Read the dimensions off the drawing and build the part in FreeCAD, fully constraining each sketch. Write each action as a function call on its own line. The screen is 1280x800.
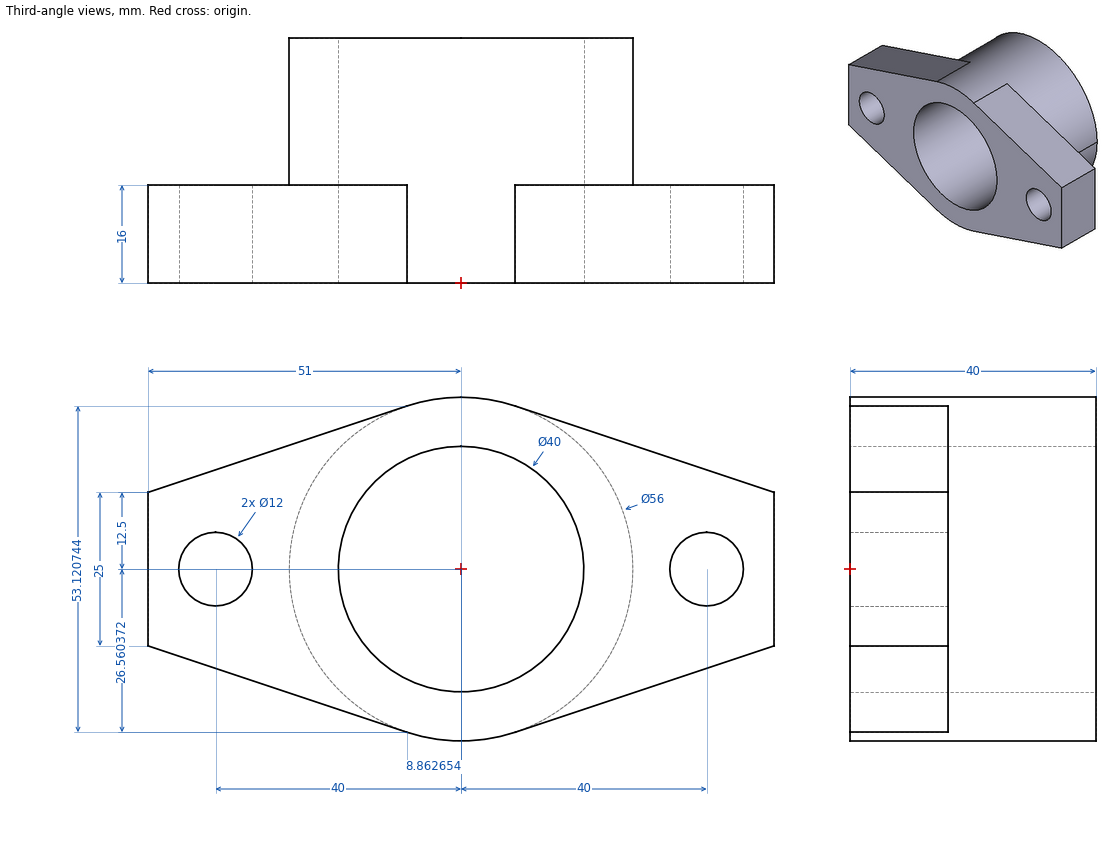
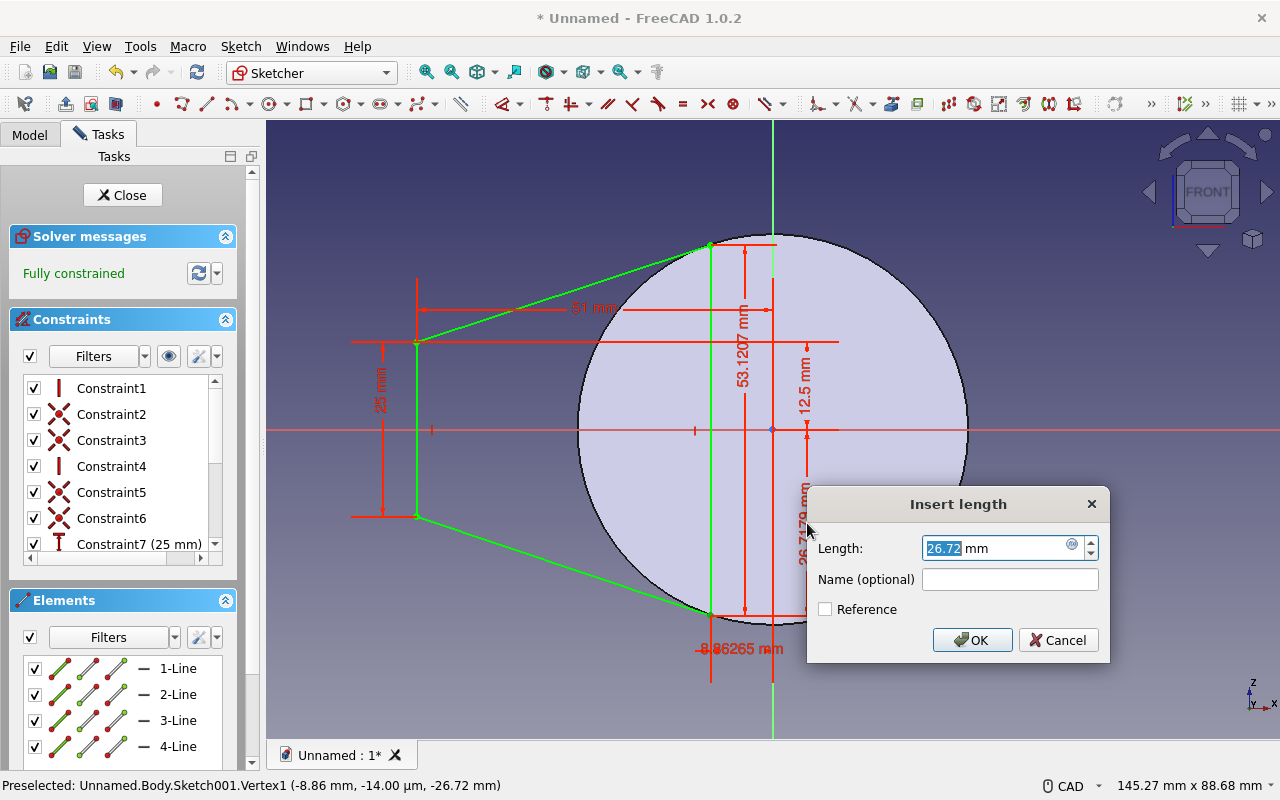
text(26.560372)
key(Return)
key(Escape)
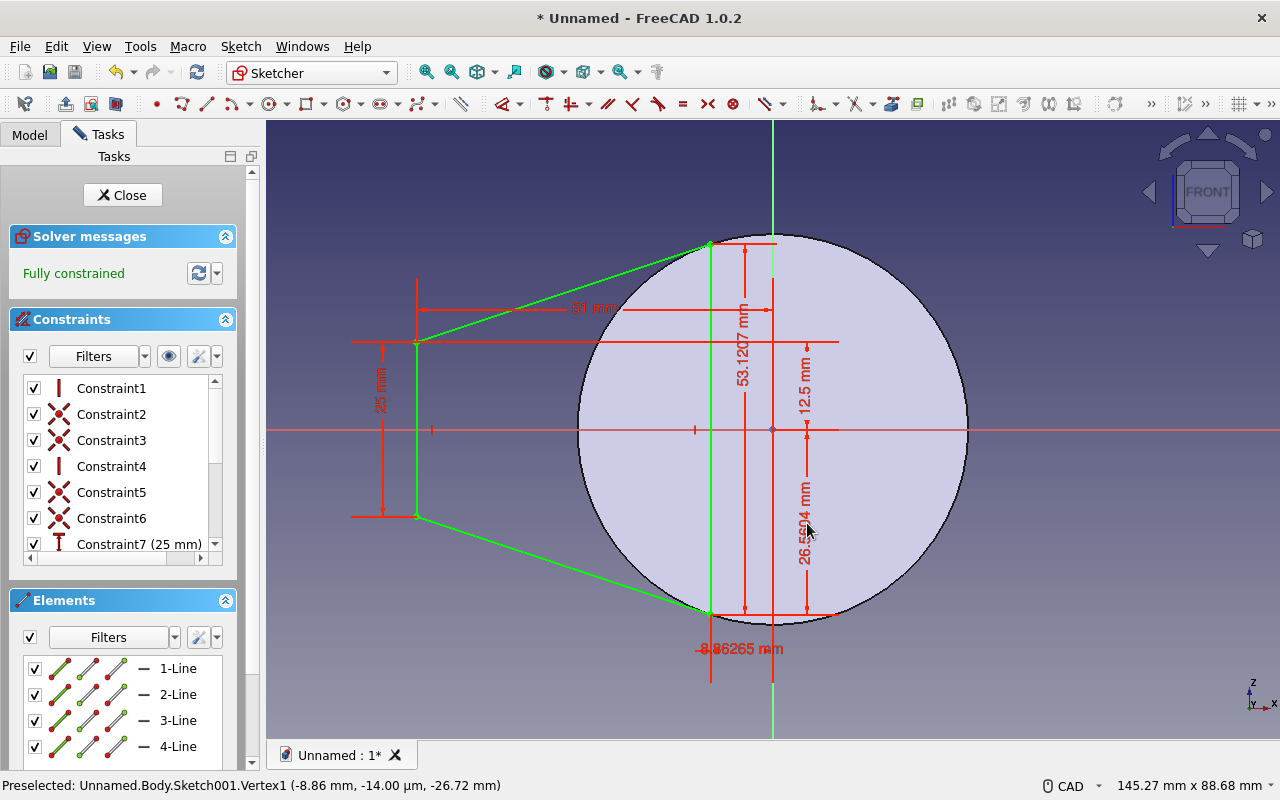
click(123, 195)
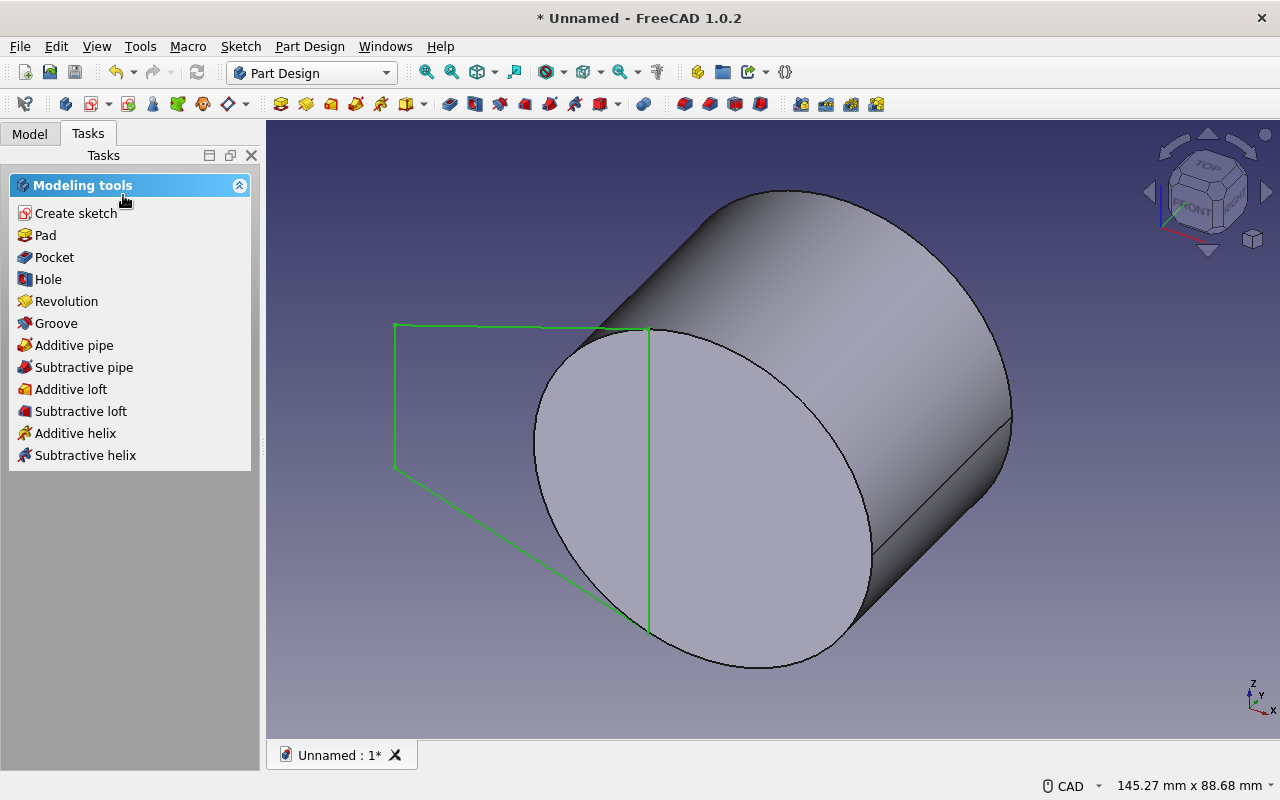
click(281, 104)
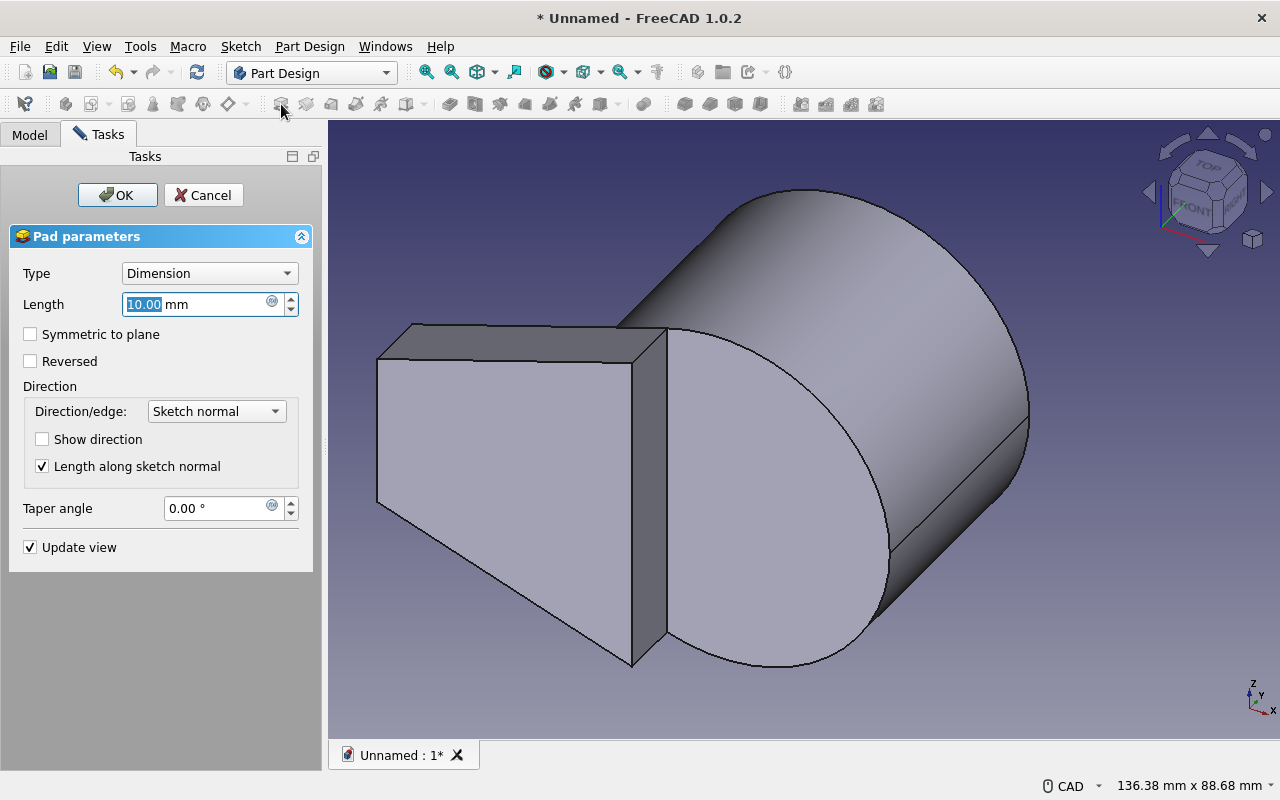
text(16)
key(Tab)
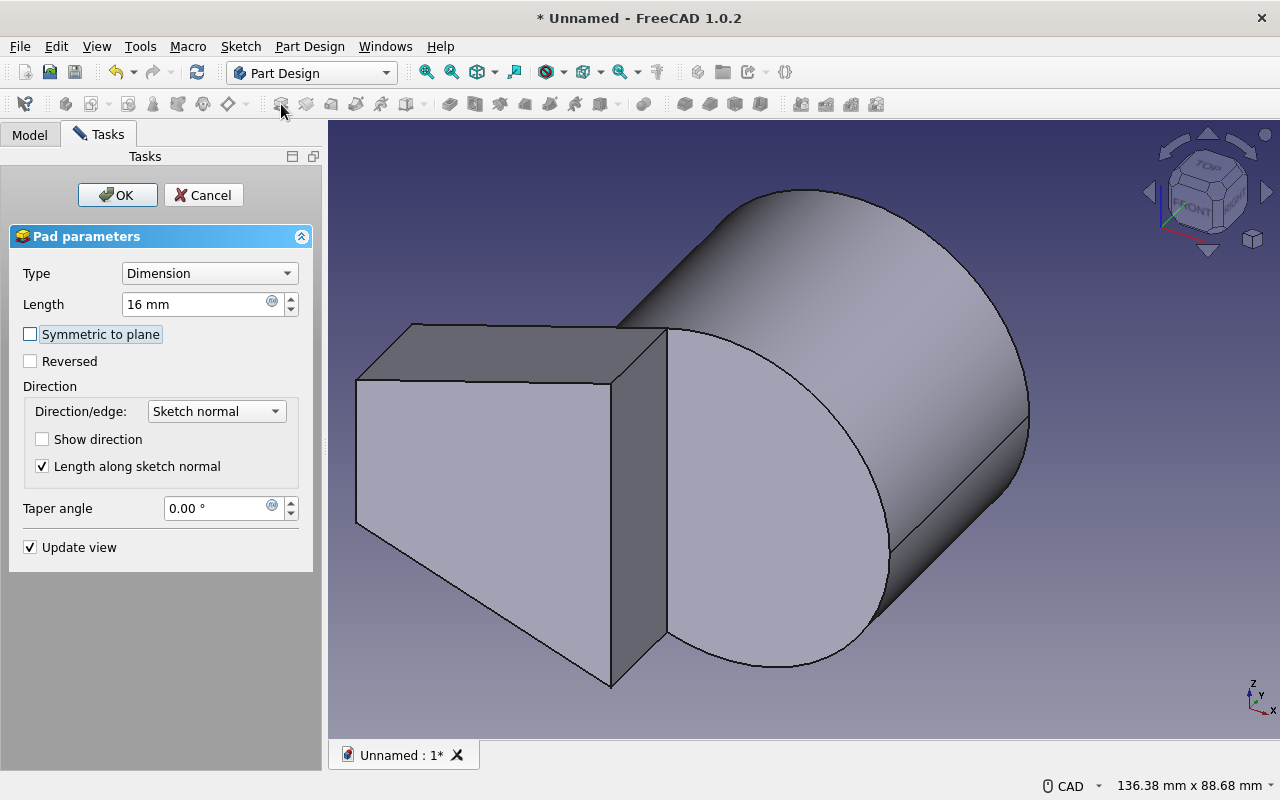
click(31, 361)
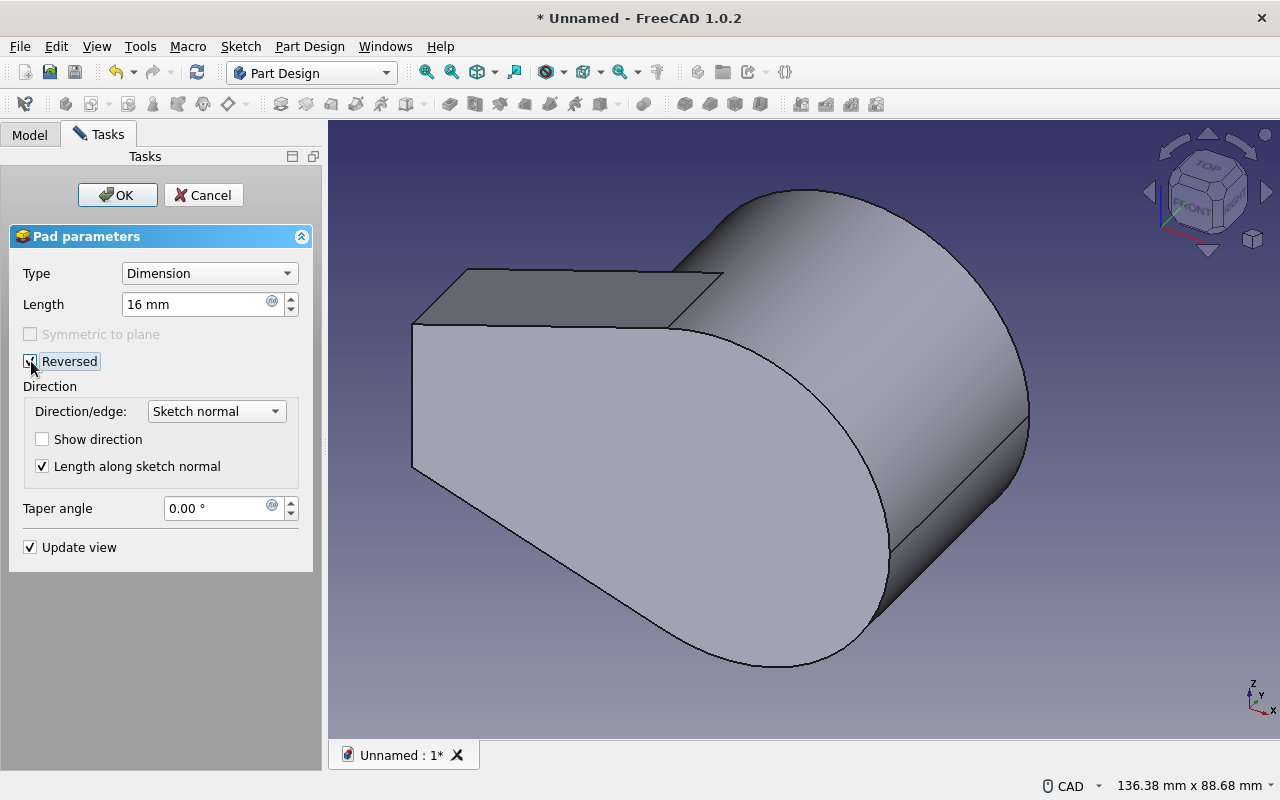
click(118, 195)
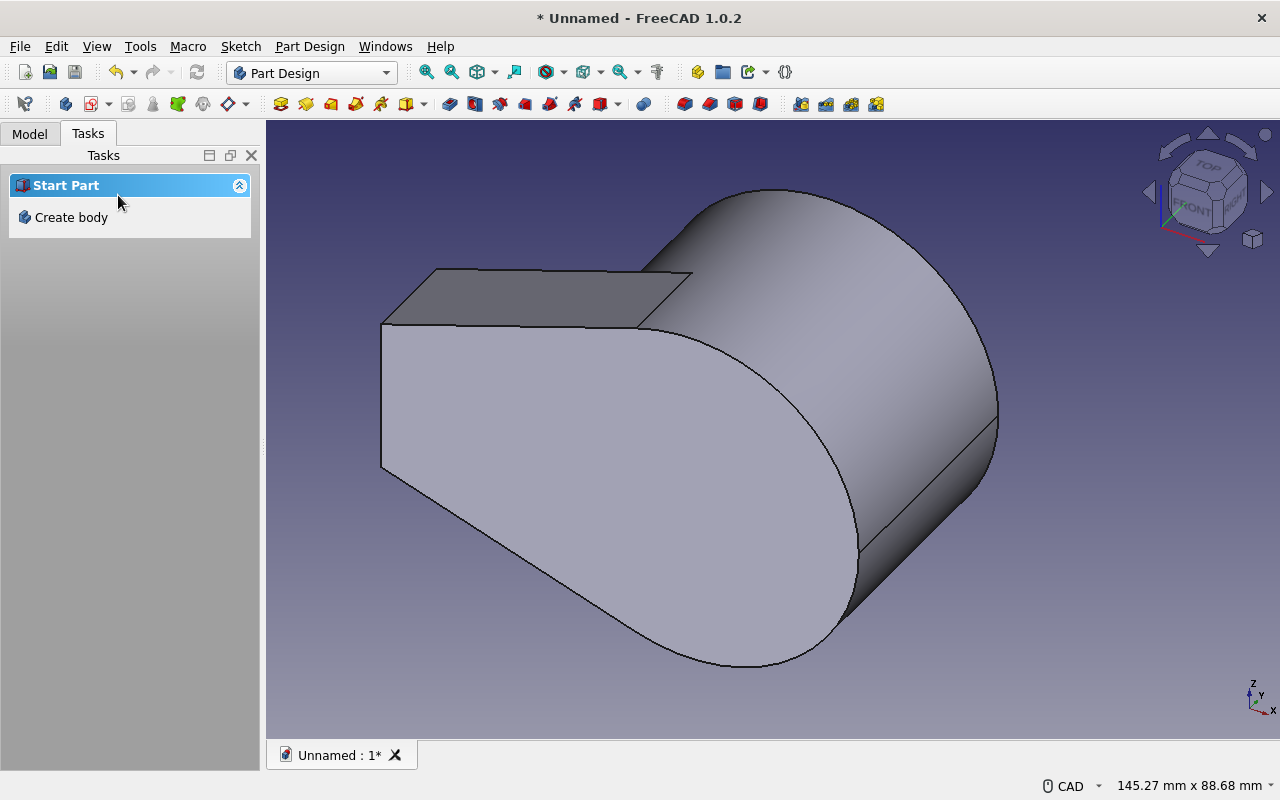
click(427, 72)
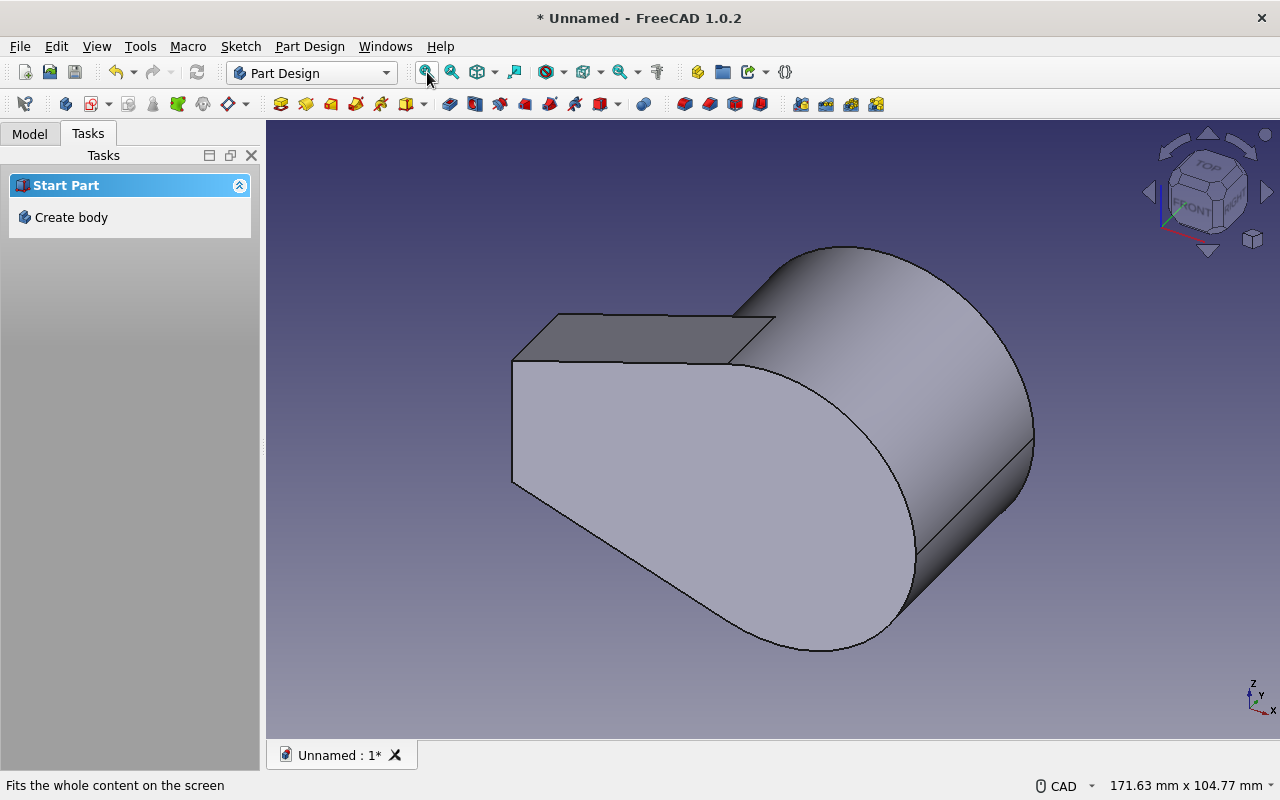
click(30, 134)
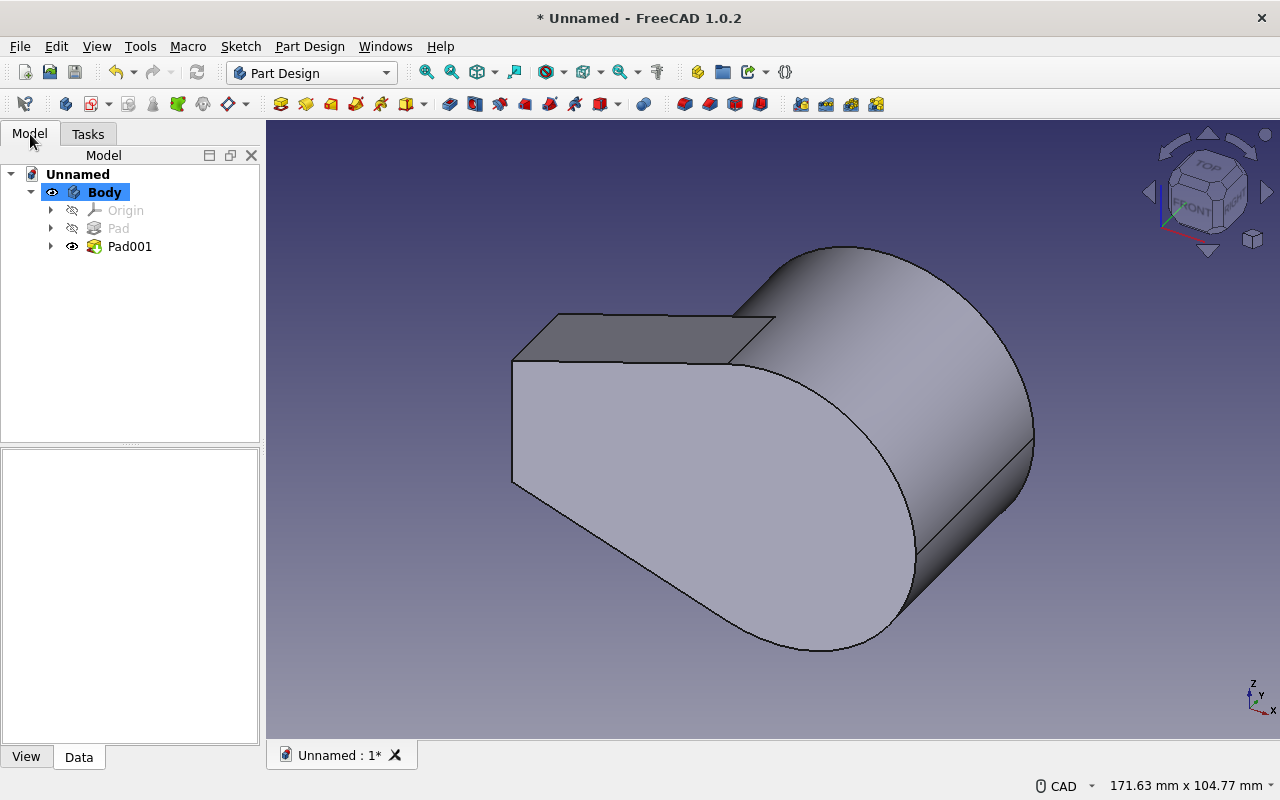
click(117, 246)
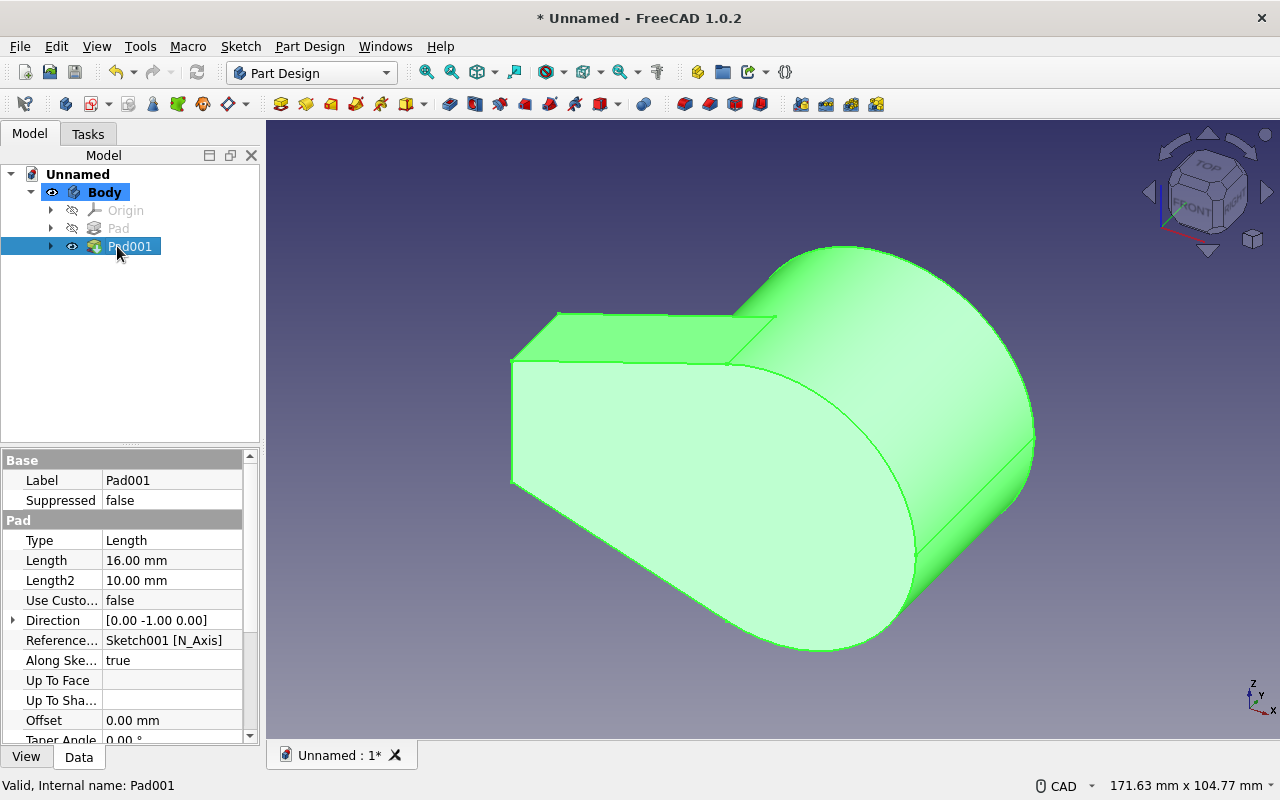
click(801, 104)